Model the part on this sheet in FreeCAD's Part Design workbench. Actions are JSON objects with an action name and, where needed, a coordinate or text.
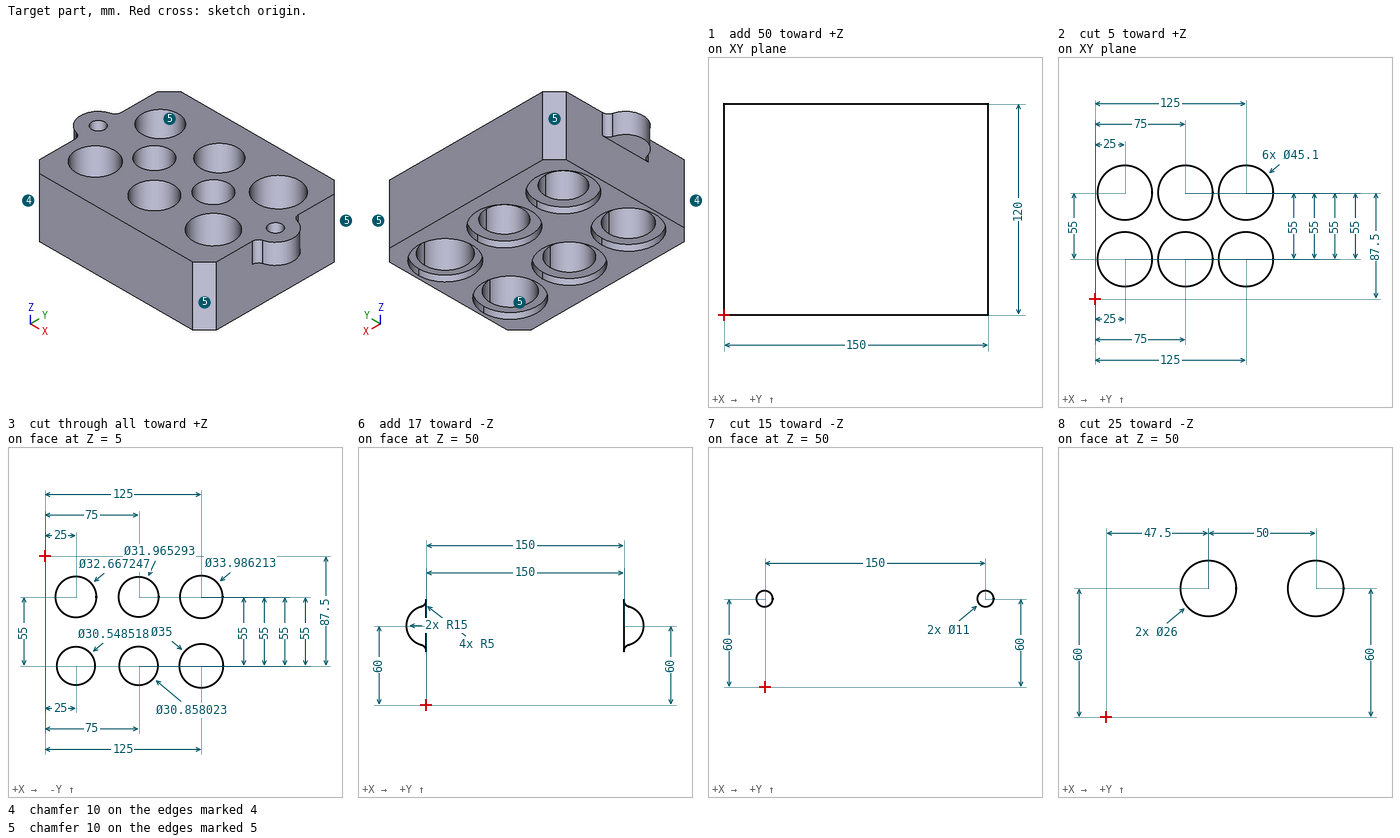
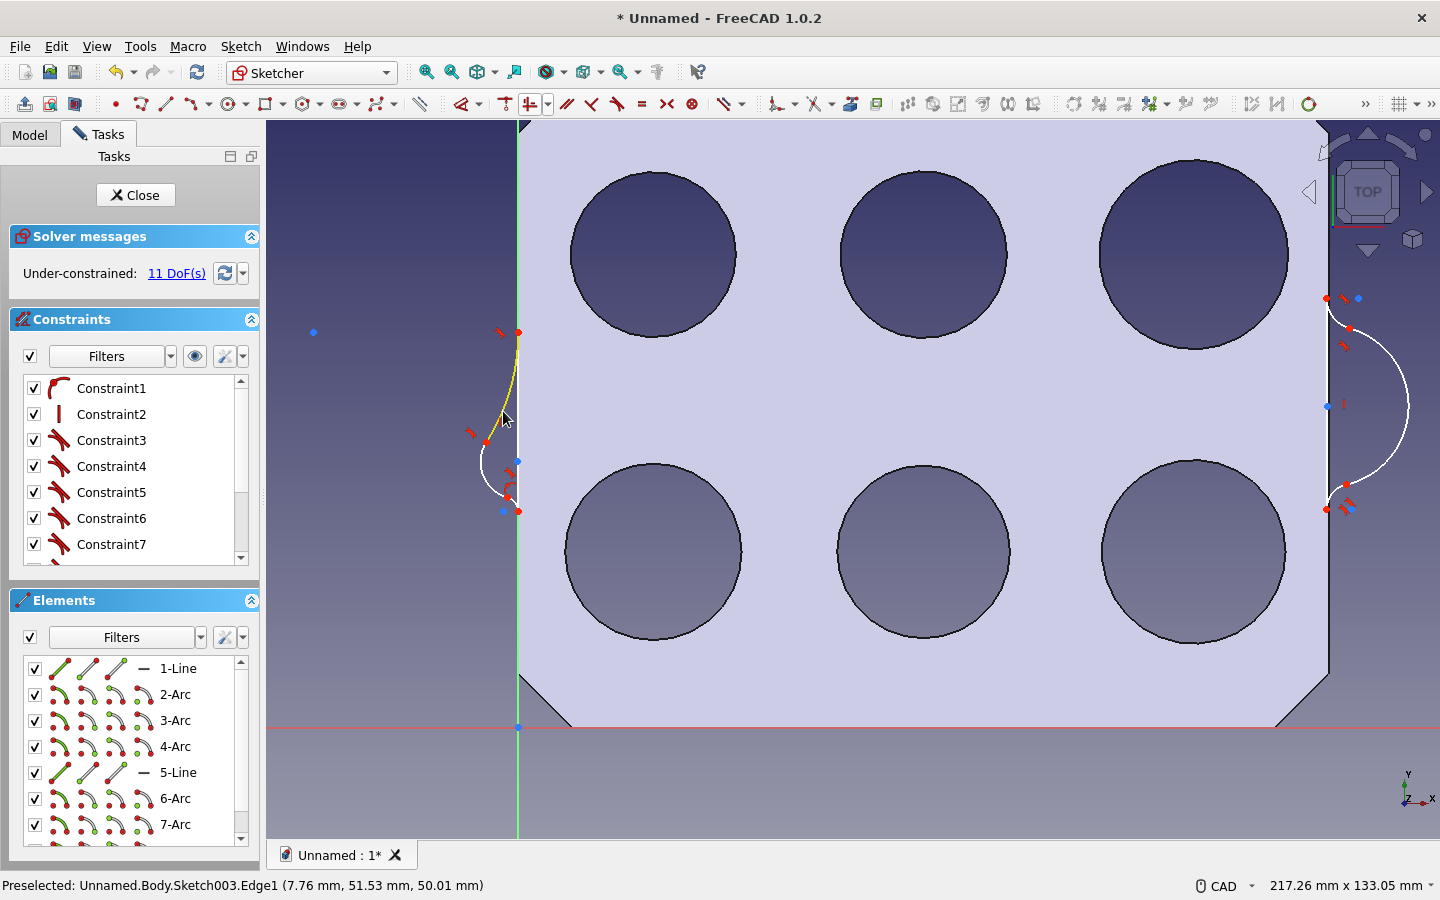
{"action": "left_click", "coordinate": [502, 411]}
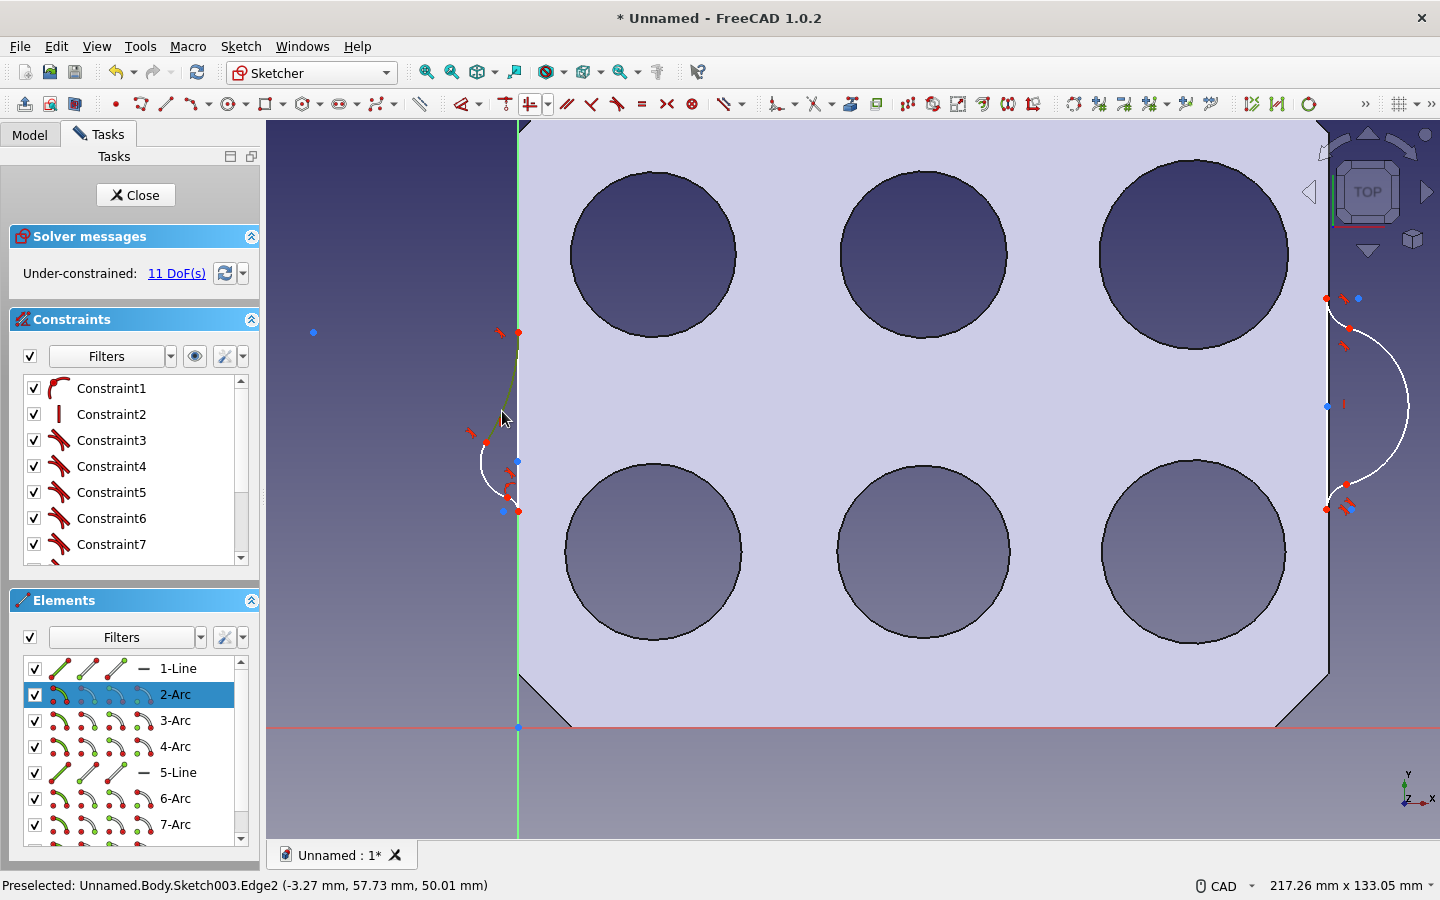
{"action": "scroll", "coordinate": [513, 500], "scroll_direction": "up", "scroll_amount": 5}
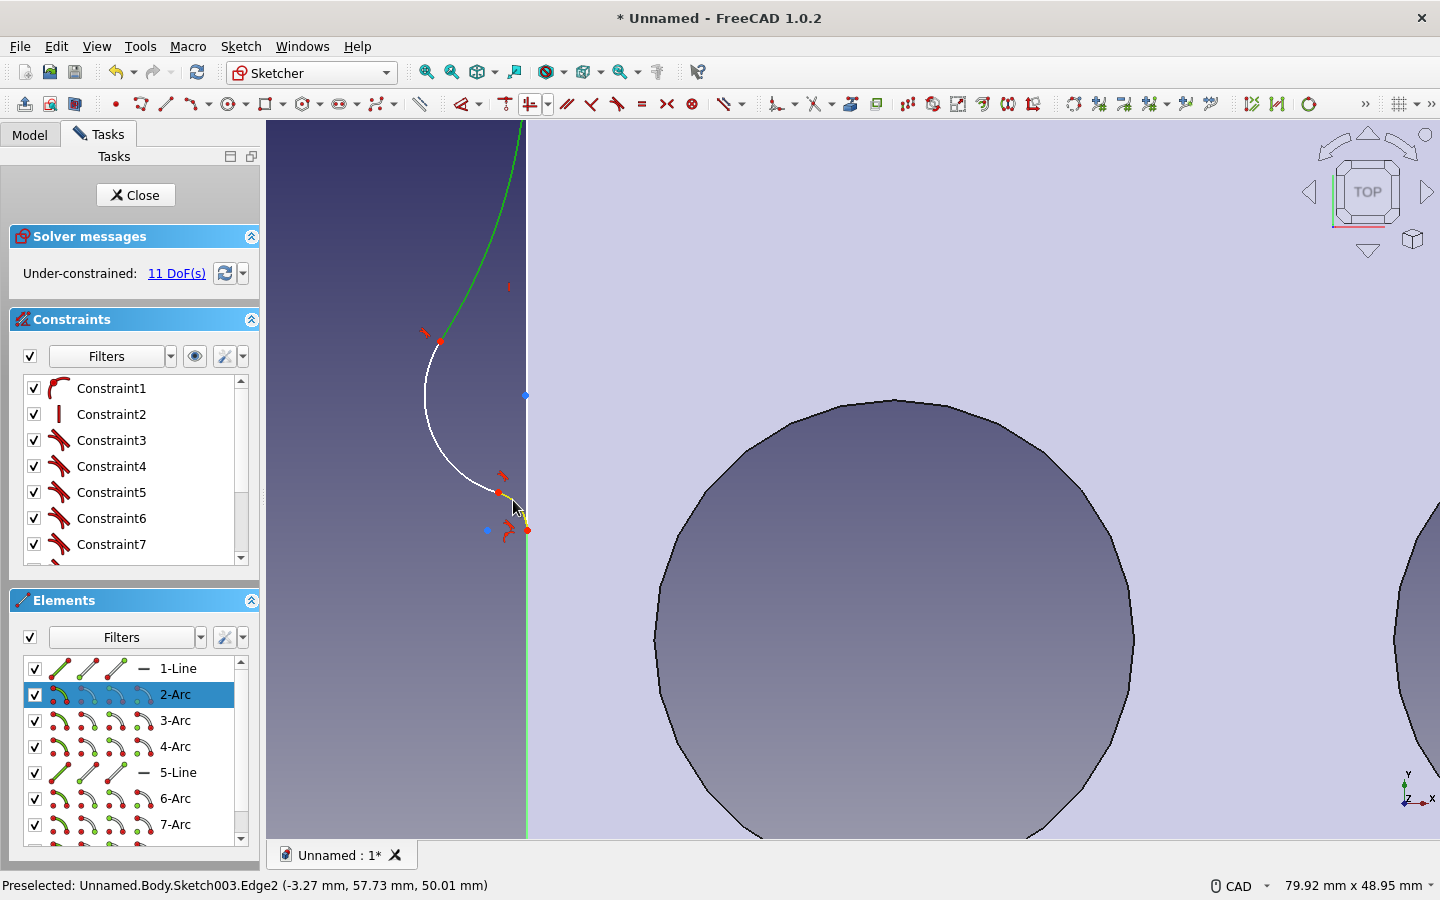
{"action": "left_click", "coordinate": [512, 500]}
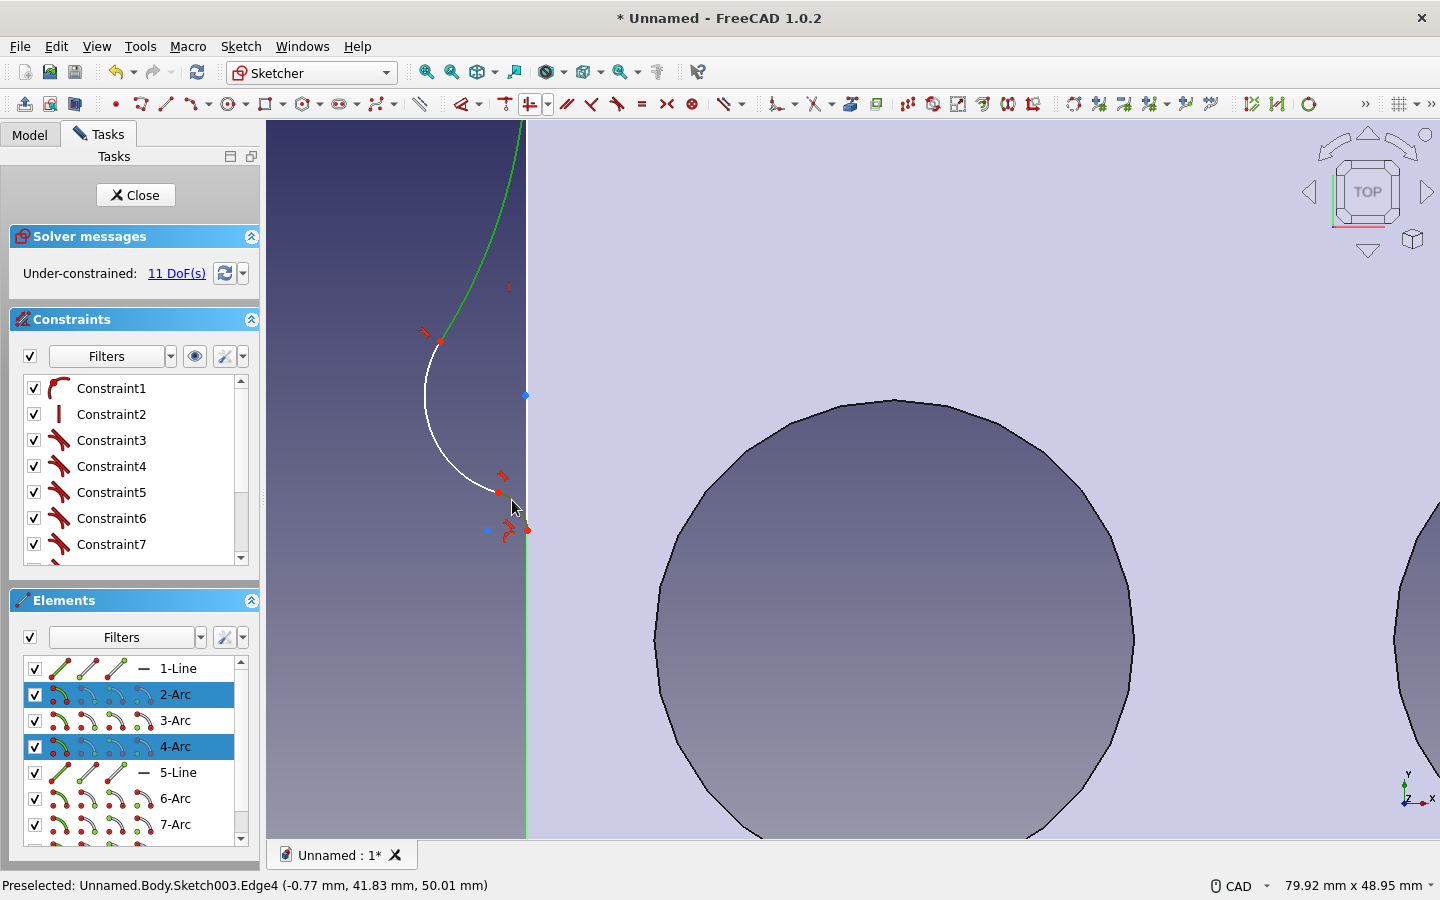
{"action": "scroll", "coordinate": [508, 461], "scroll_direction": "down", "scroll_amount": 7}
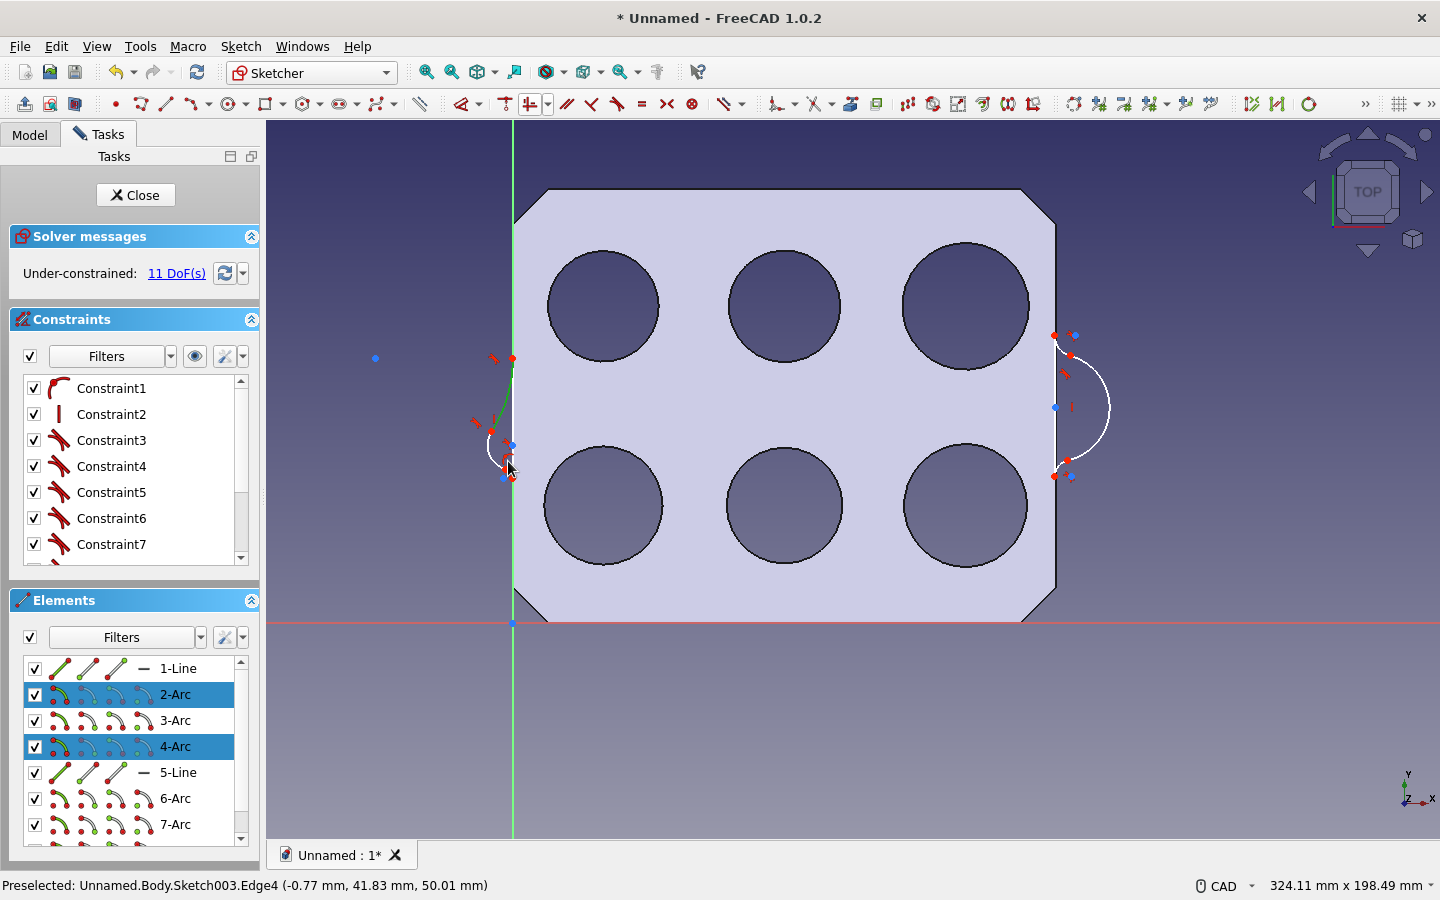
{"action": "scroll", "coordinate": [1062, 463], "scroll_direction": "up", "scroll_amount": 4}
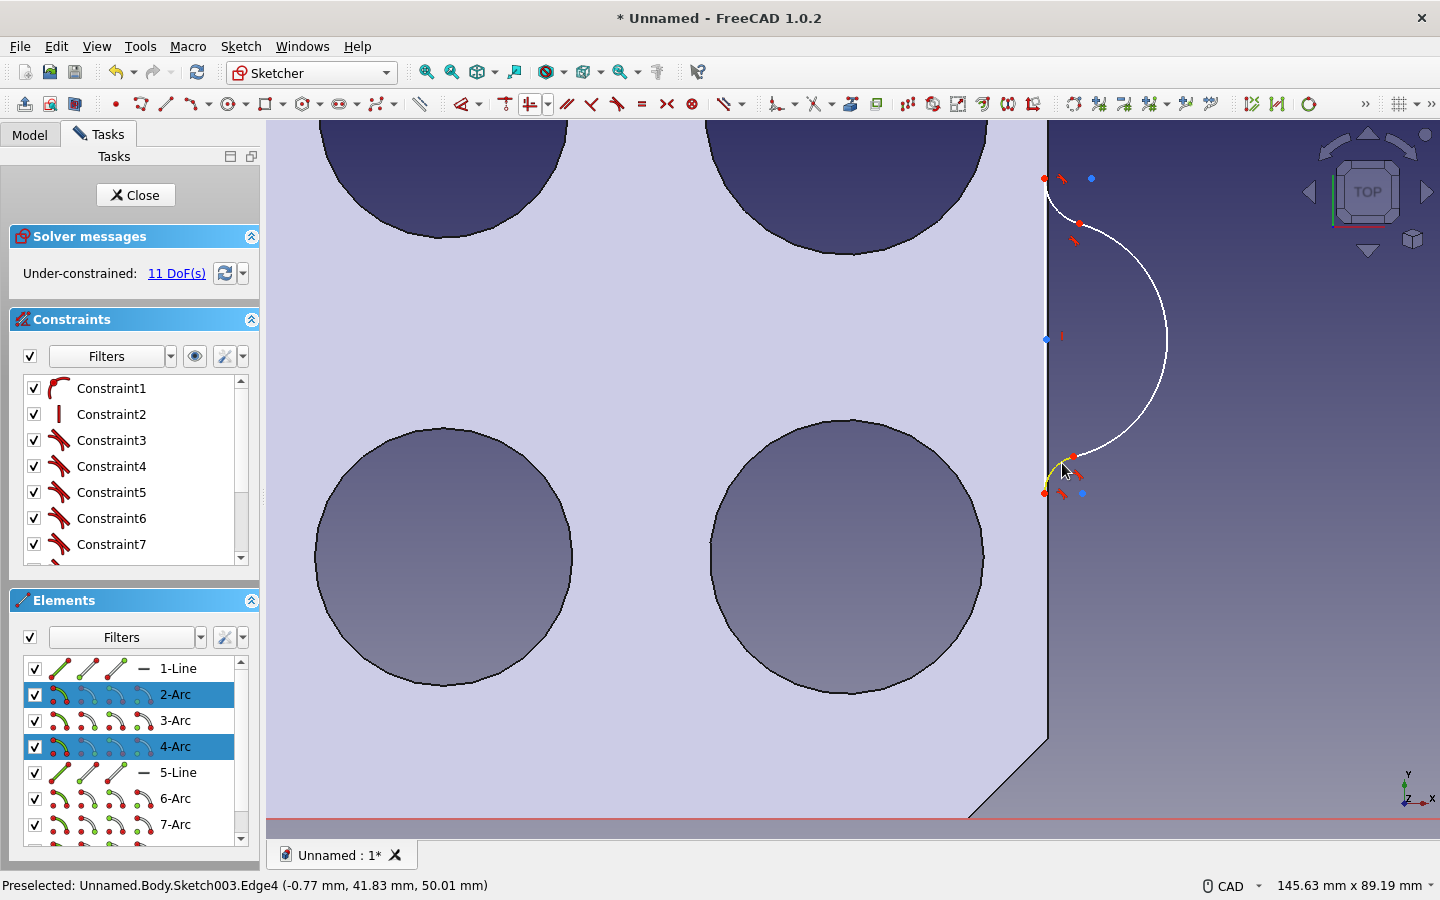
{"action": "left_click", "coordinate": [1060, 463]}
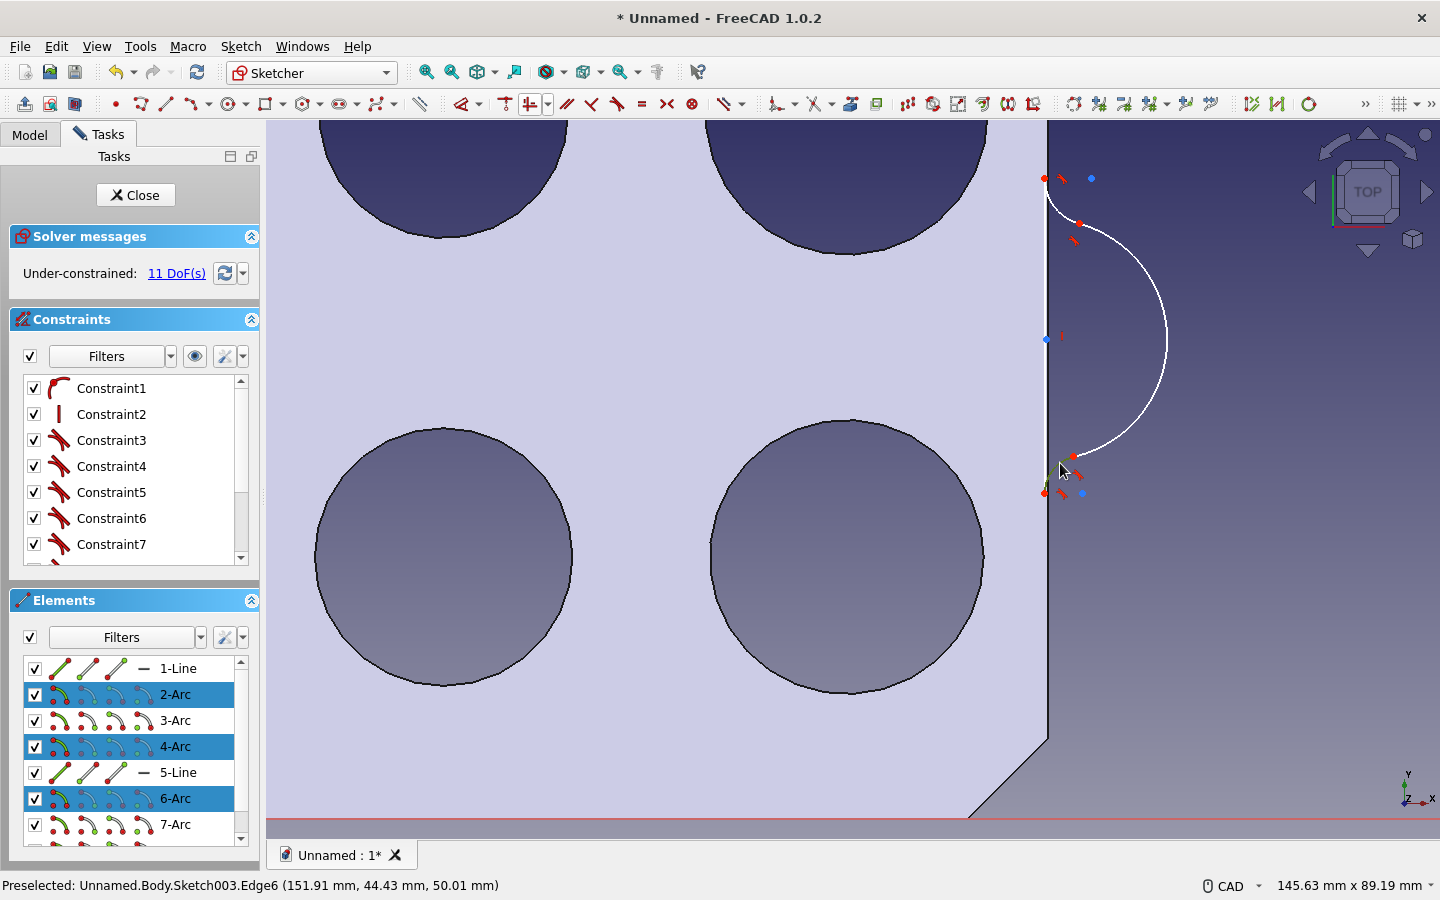
{"action": "left_click", "coordinate": [1063, 215]}